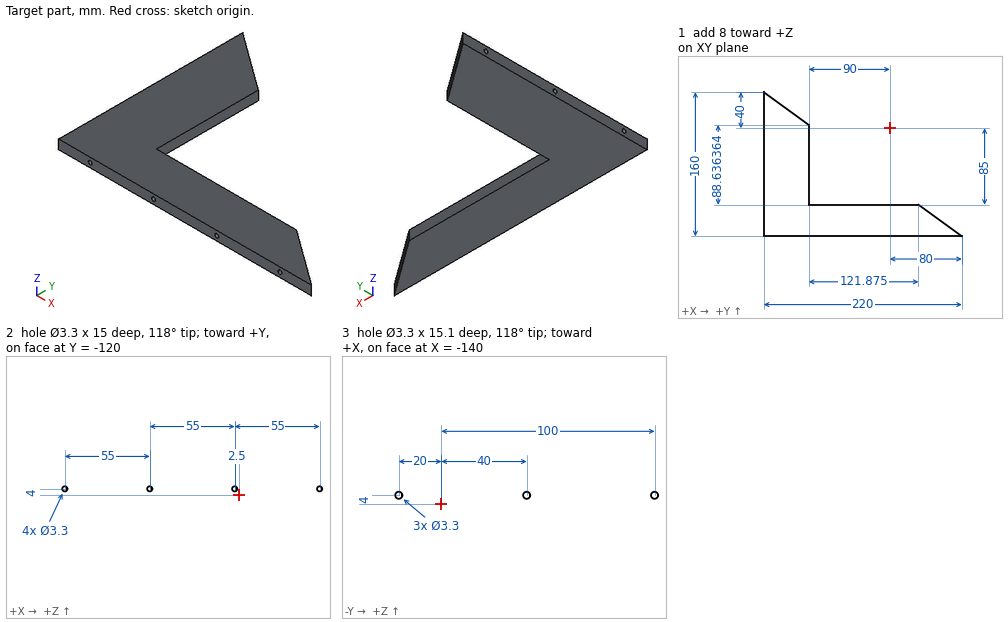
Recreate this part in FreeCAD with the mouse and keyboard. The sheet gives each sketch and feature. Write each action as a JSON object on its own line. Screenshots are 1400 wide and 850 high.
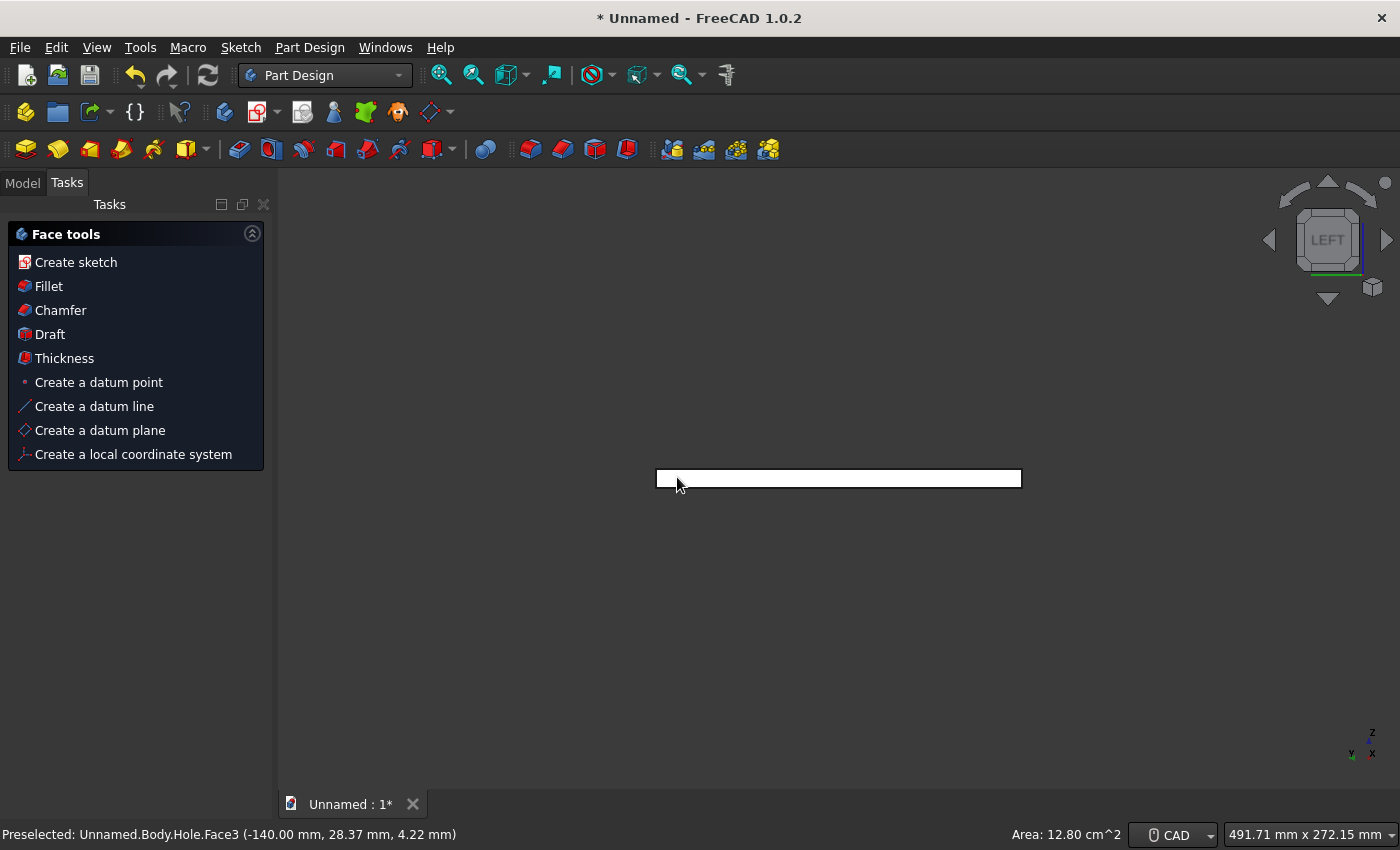
{"action": "left_click", "coordinate": [258, 112]}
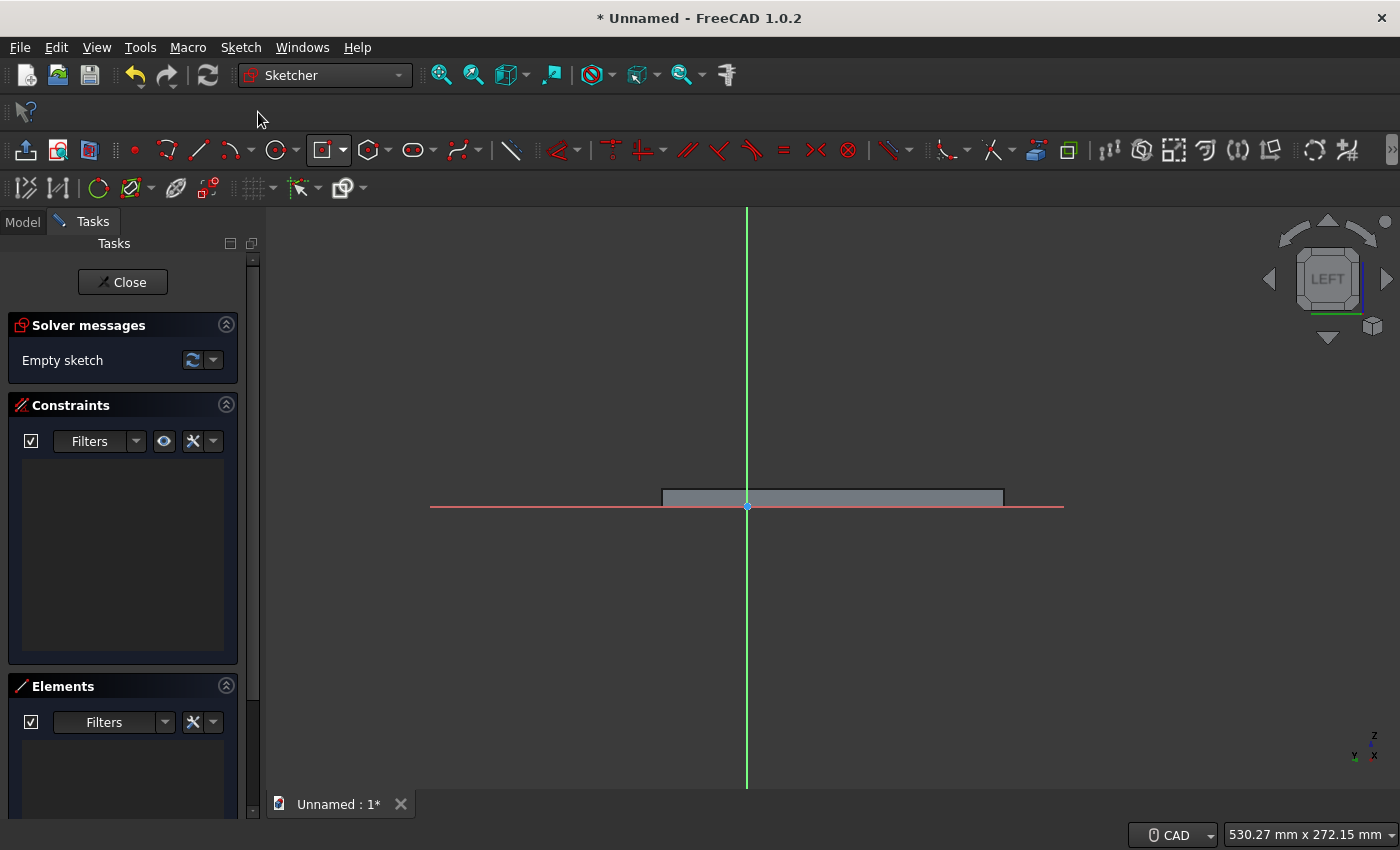
{"action": "scroll", "coordinate": [873, 502], "scroll_direction": "up", "scroll_amount": 5}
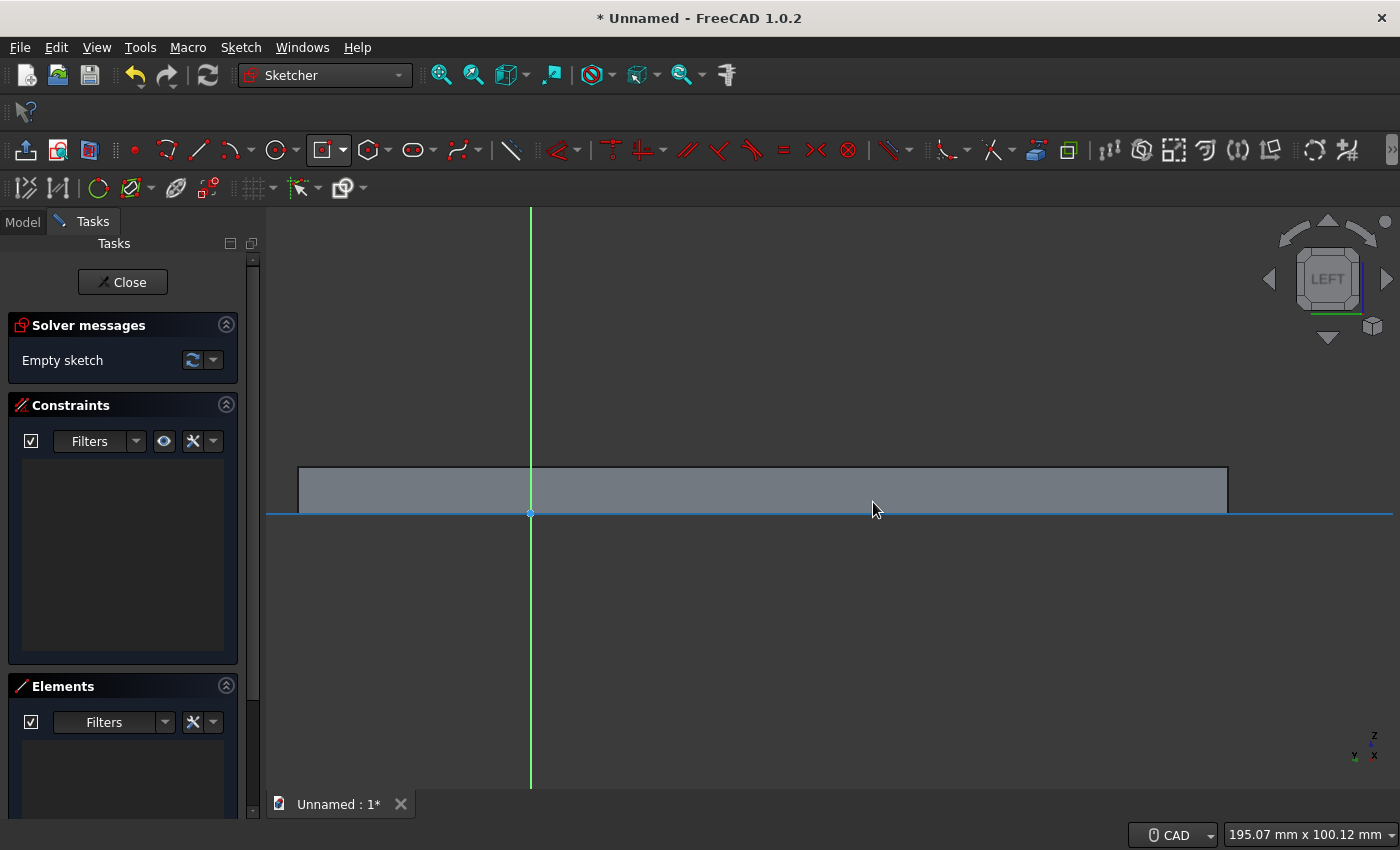
{"action": "key", "text": "g c"}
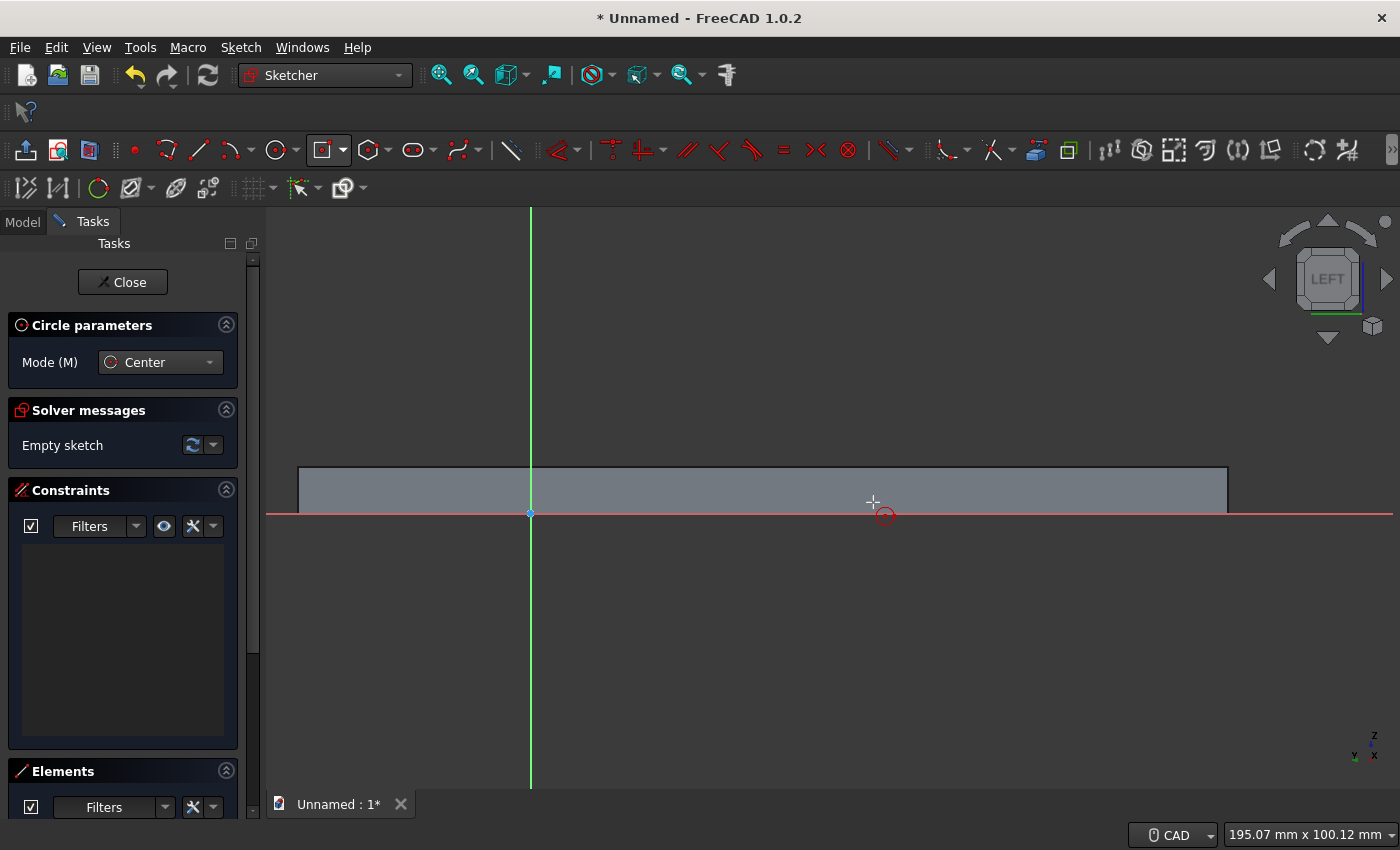
{"action": "scroll", "coordinate": [415, 490], "scroll_direction": "up", "scroll_amount": 5}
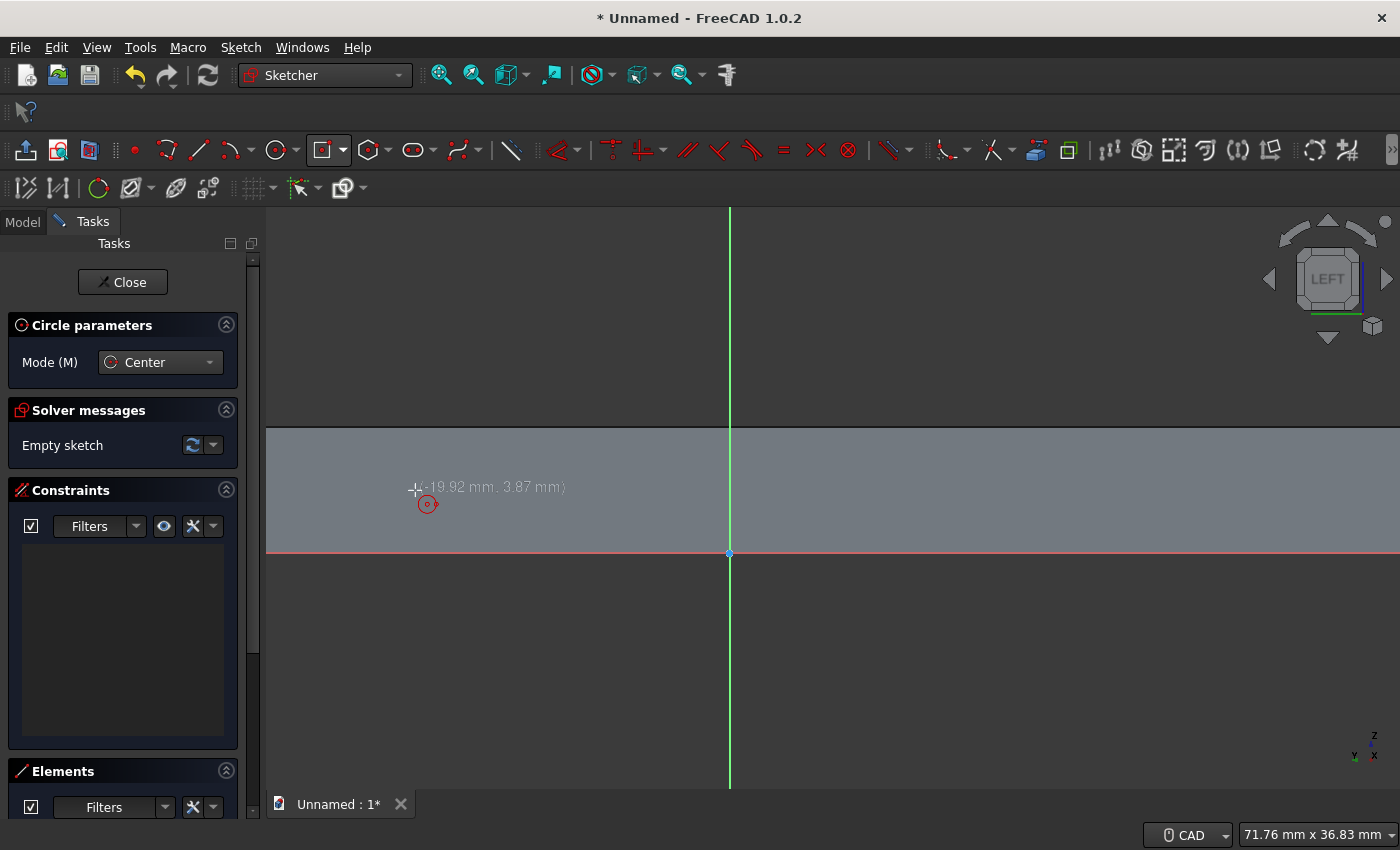
{"action": "left_click", "coordinate": [414, 490]}
{"action": "left_click", "coordinate": [432, 471]}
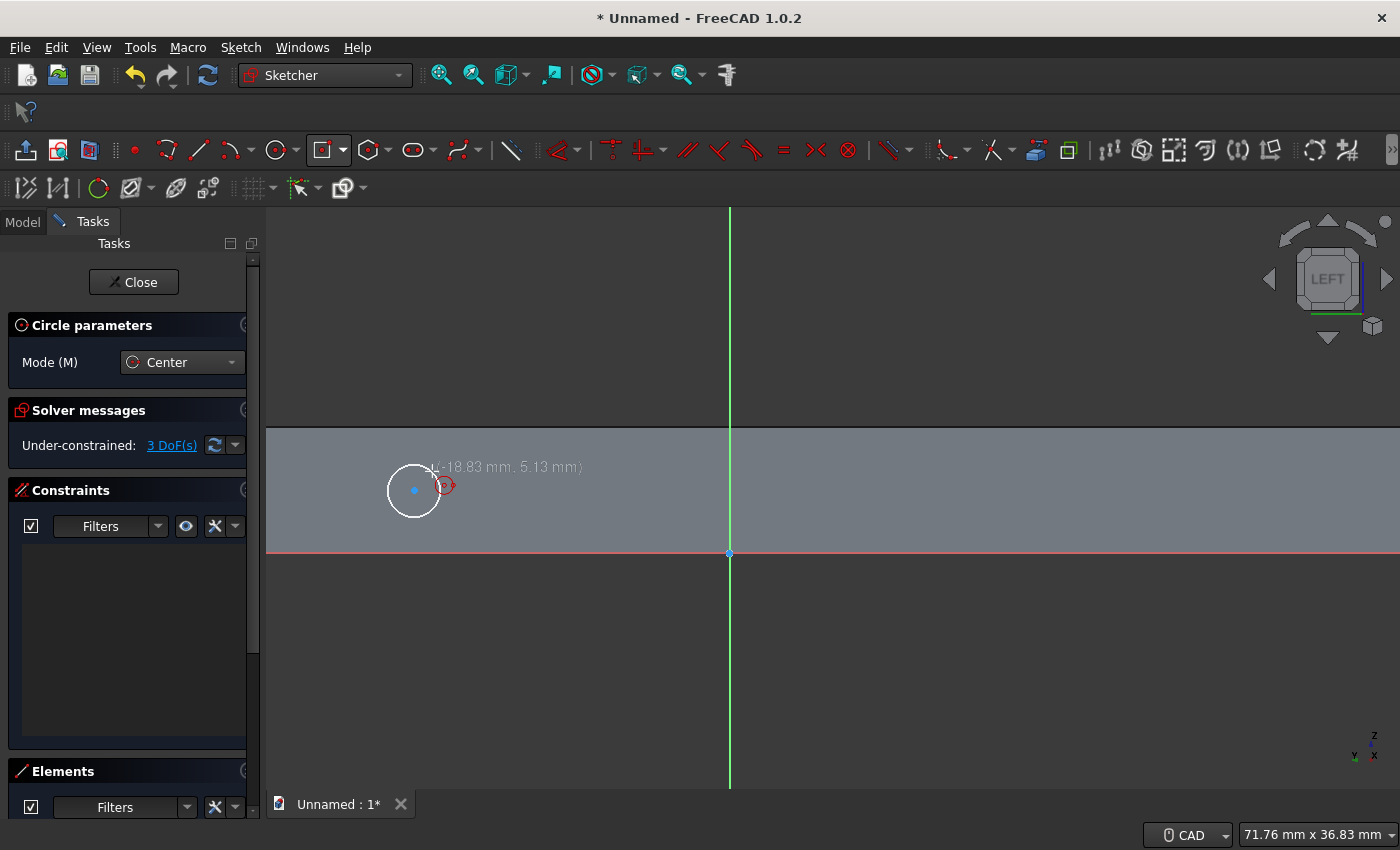
{"action": "scroll", "coordinate": [417, 492], "scroll_direction": "down", "scroll_amount": 5}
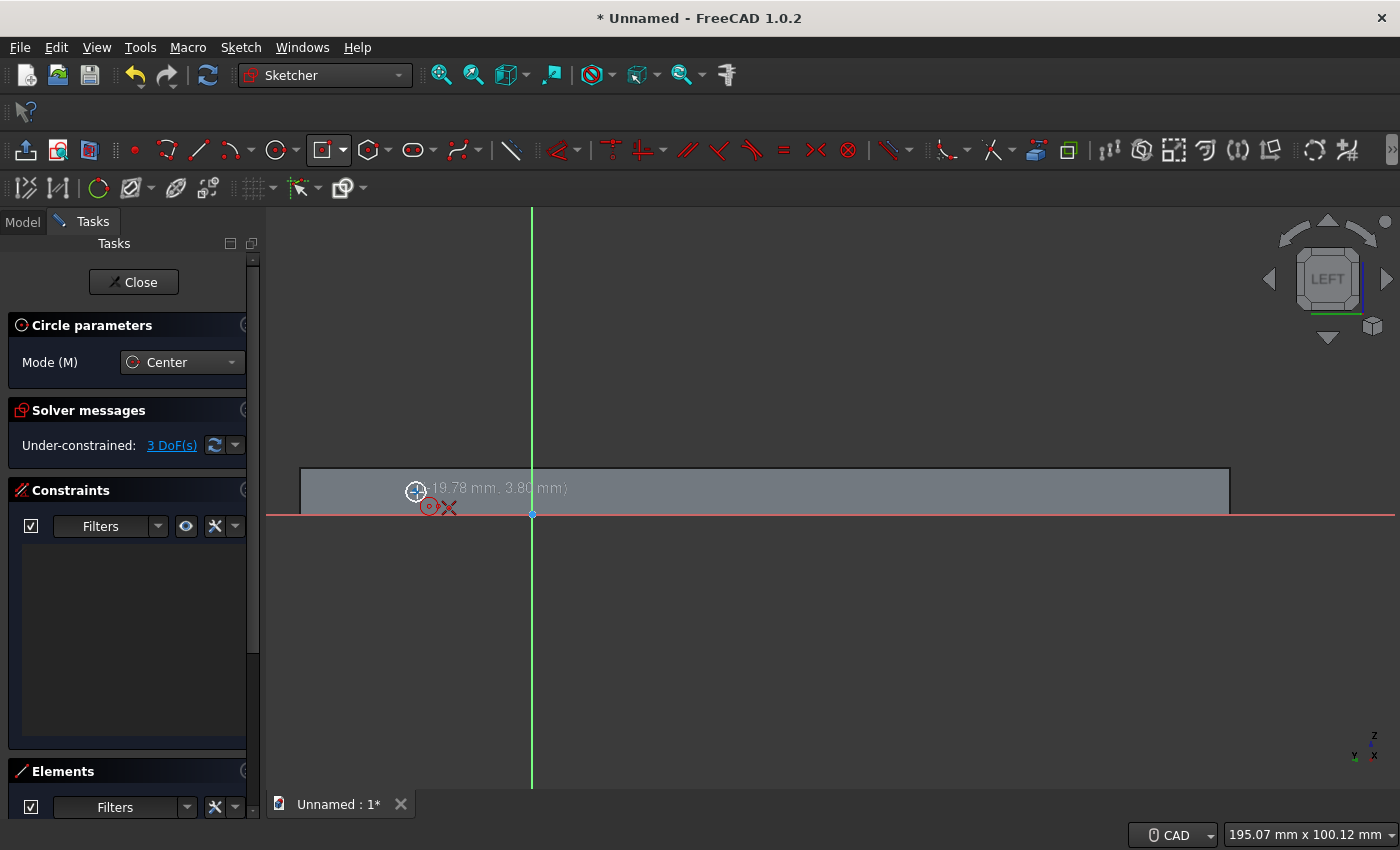
{"action": "scroll", "coordinate": [765, 492], "scroll_direction": "up", "scroll_amount": 5}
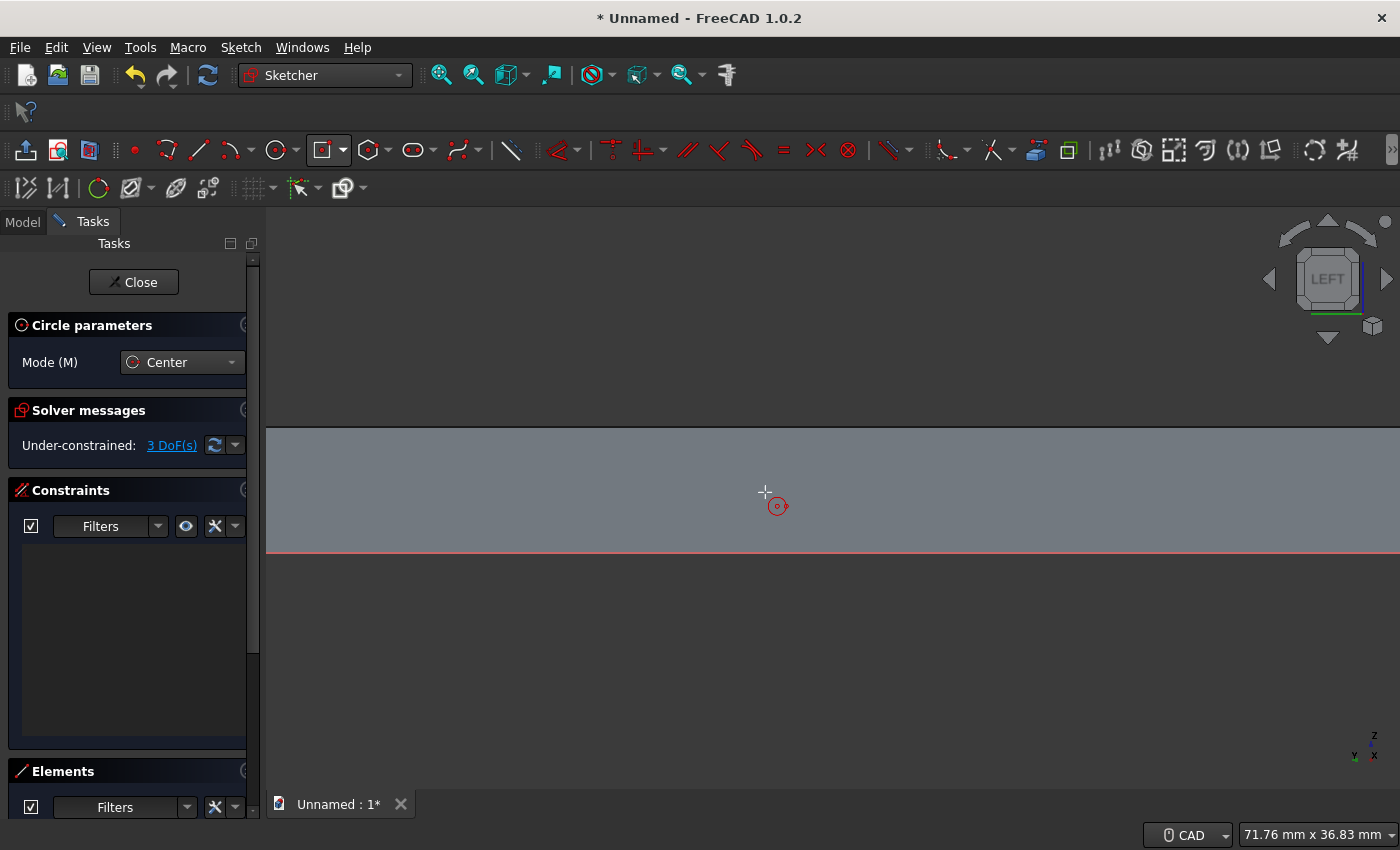
{"action": "left_click", "coordinate": [763, 490]}
{"action": "left_click", "coordinate": [782, 471]}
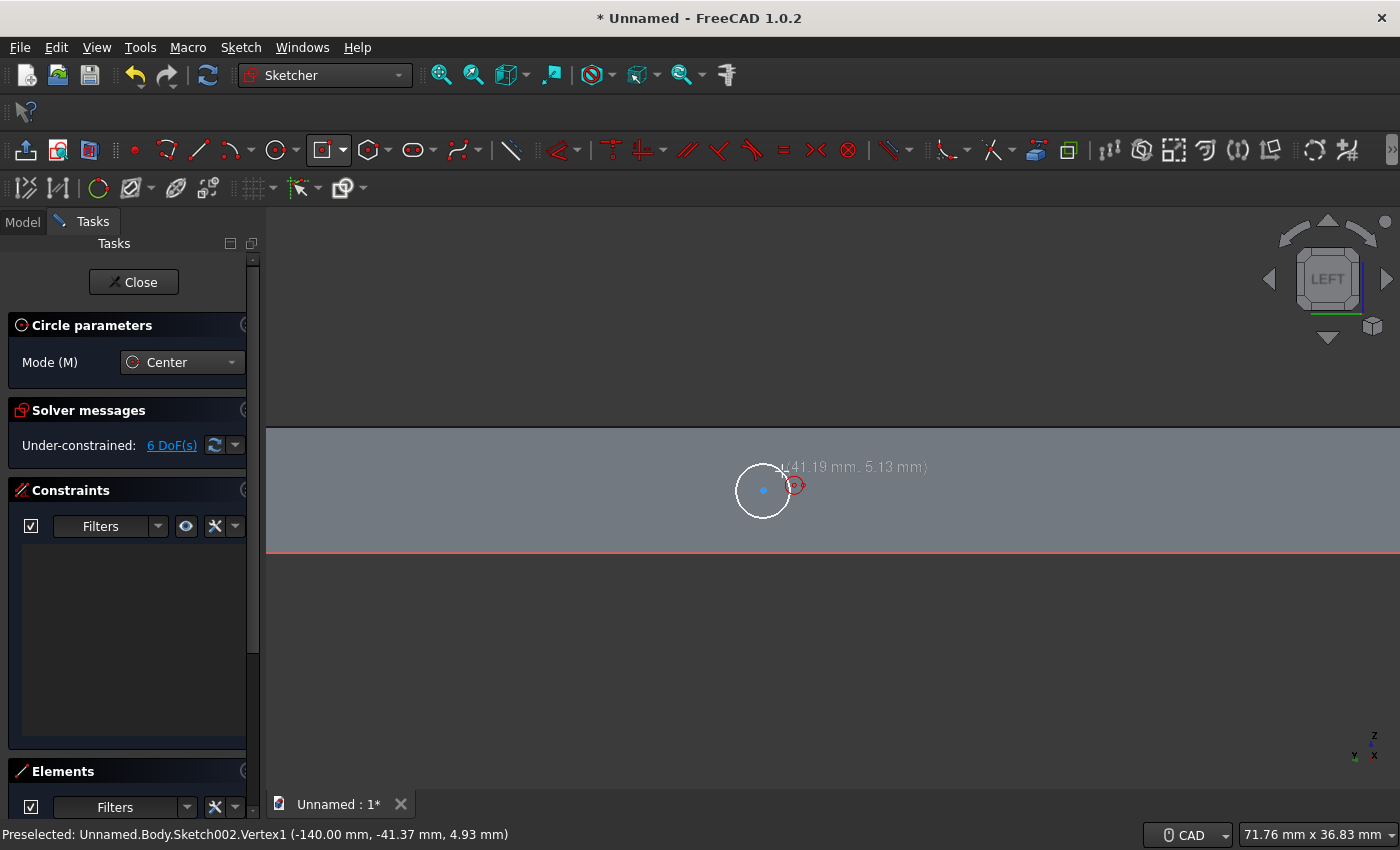
{"action": "scroll", "coordinate": [765, 492], "scroll_direction": "down", "scroll_amount": 5}